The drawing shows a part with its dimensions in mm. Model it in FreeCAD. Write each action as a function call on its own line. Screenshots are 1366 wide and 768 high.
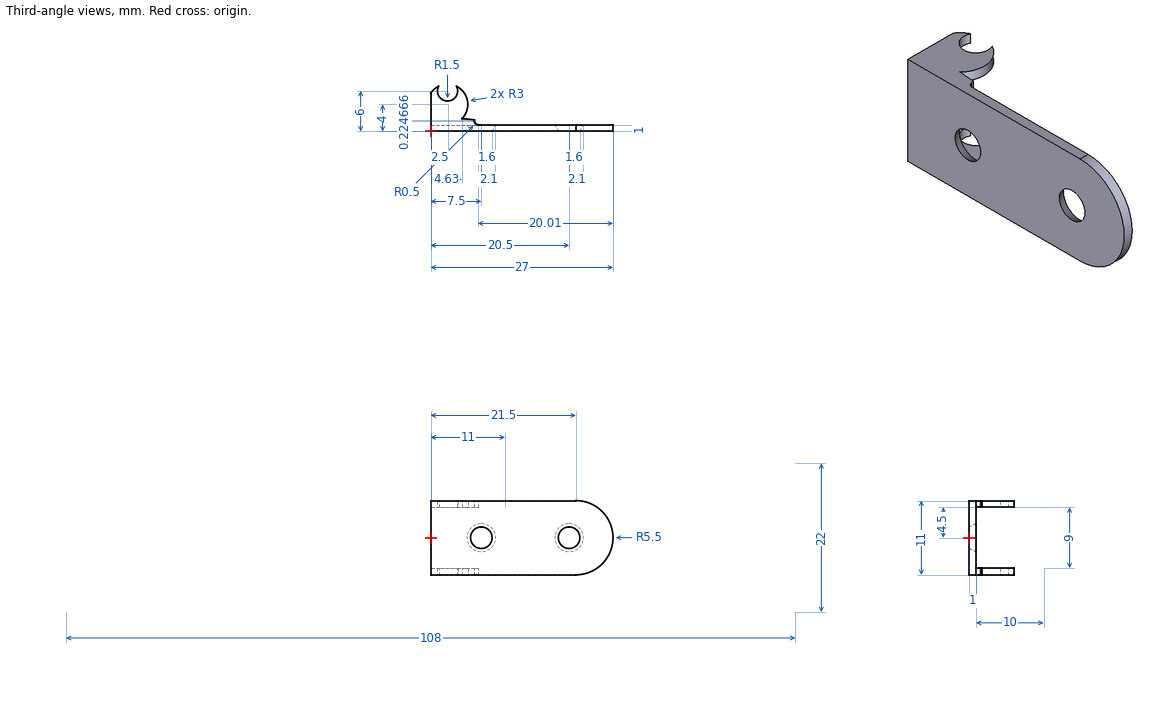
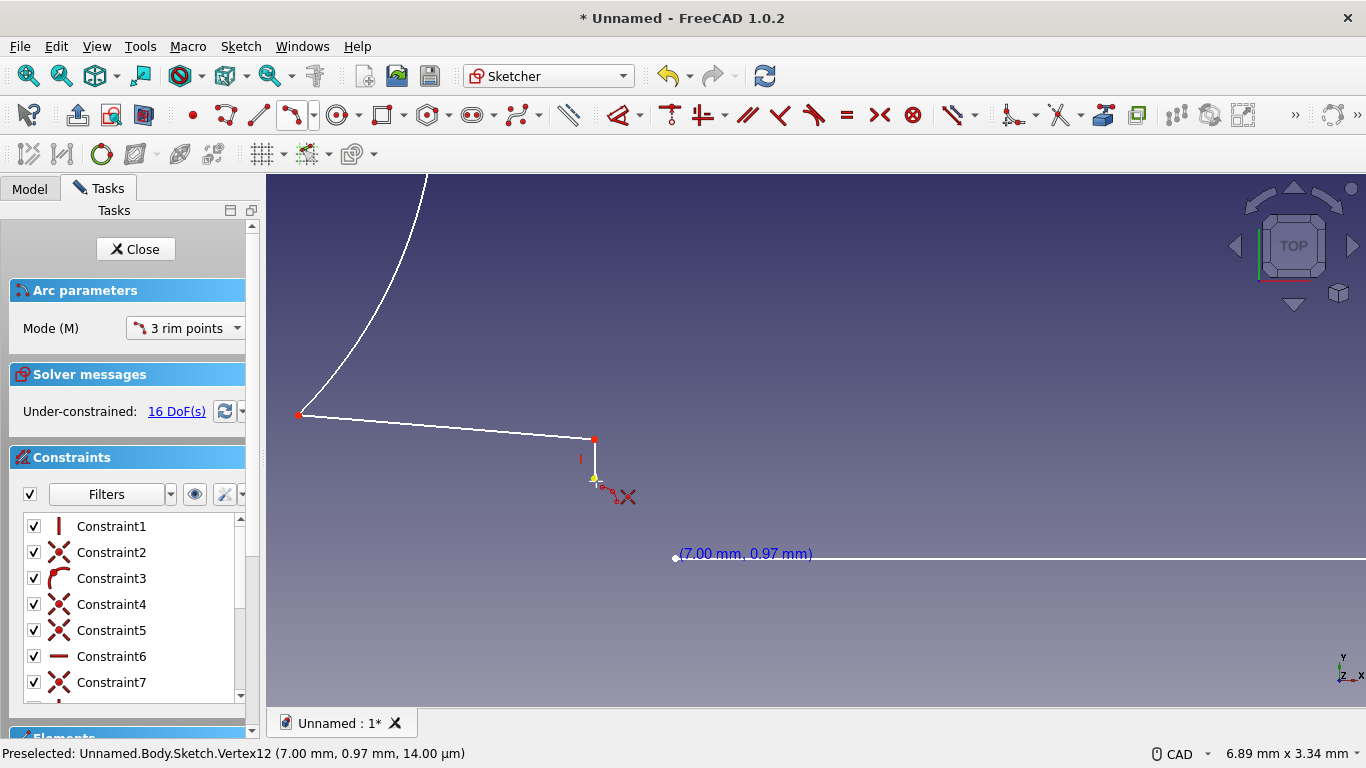
click(595, 478)
click(618, 531)
key(Escape)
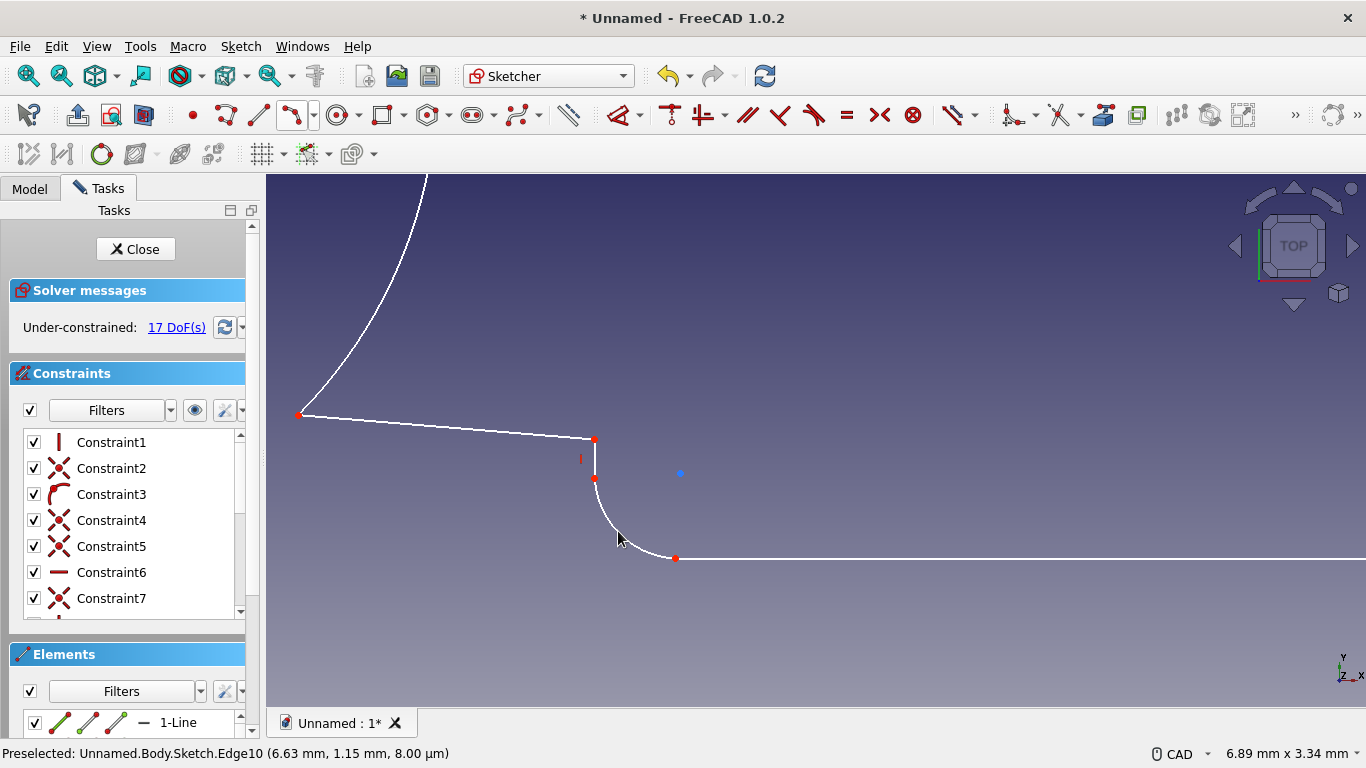
click(595, 467)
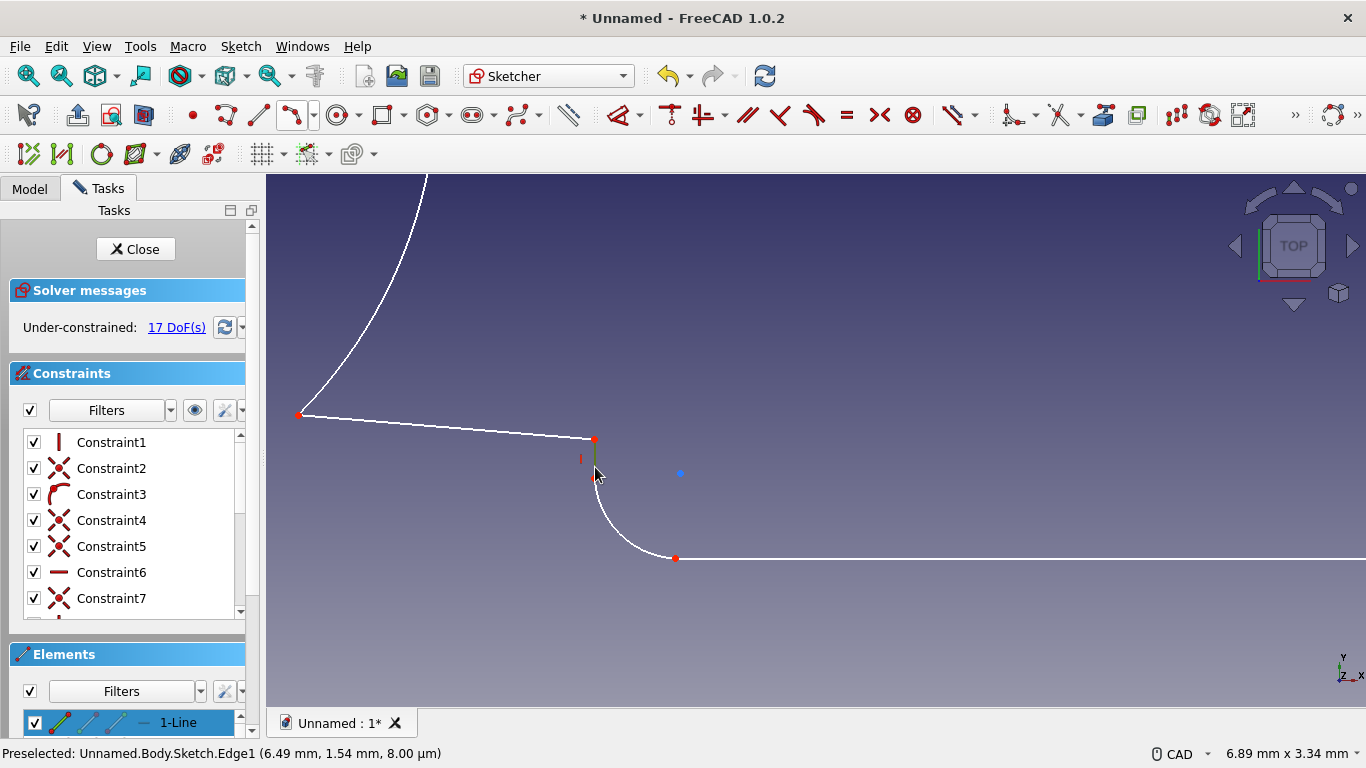
click(605, 514)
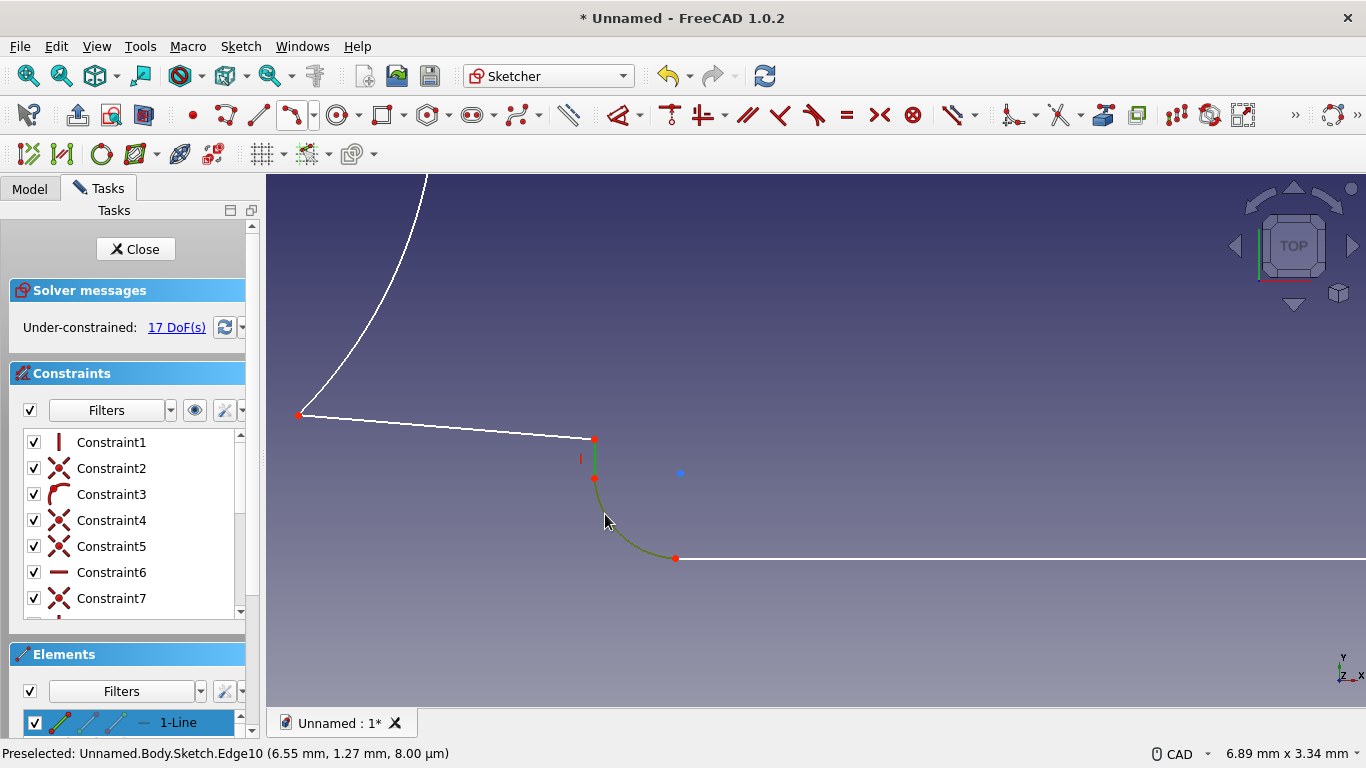
key(t)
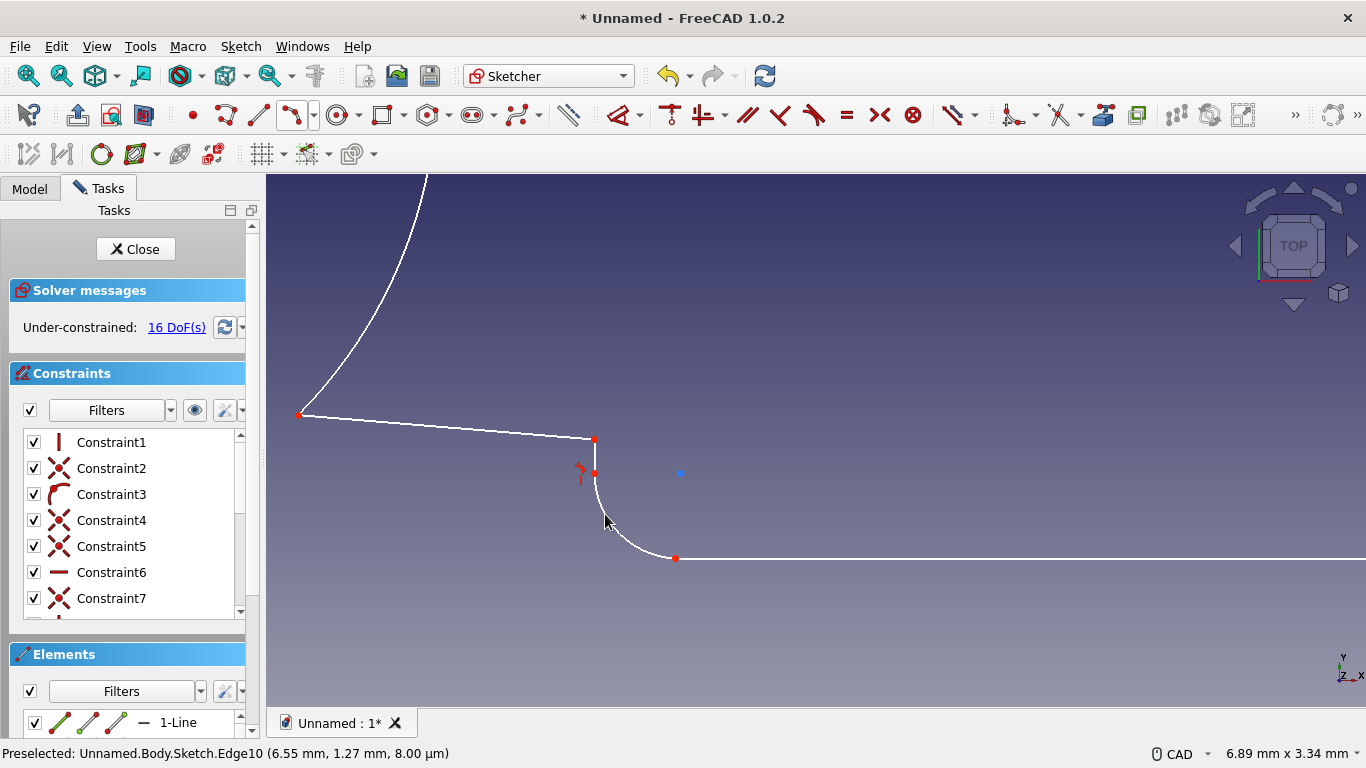
scroll(596, 481, down, 10)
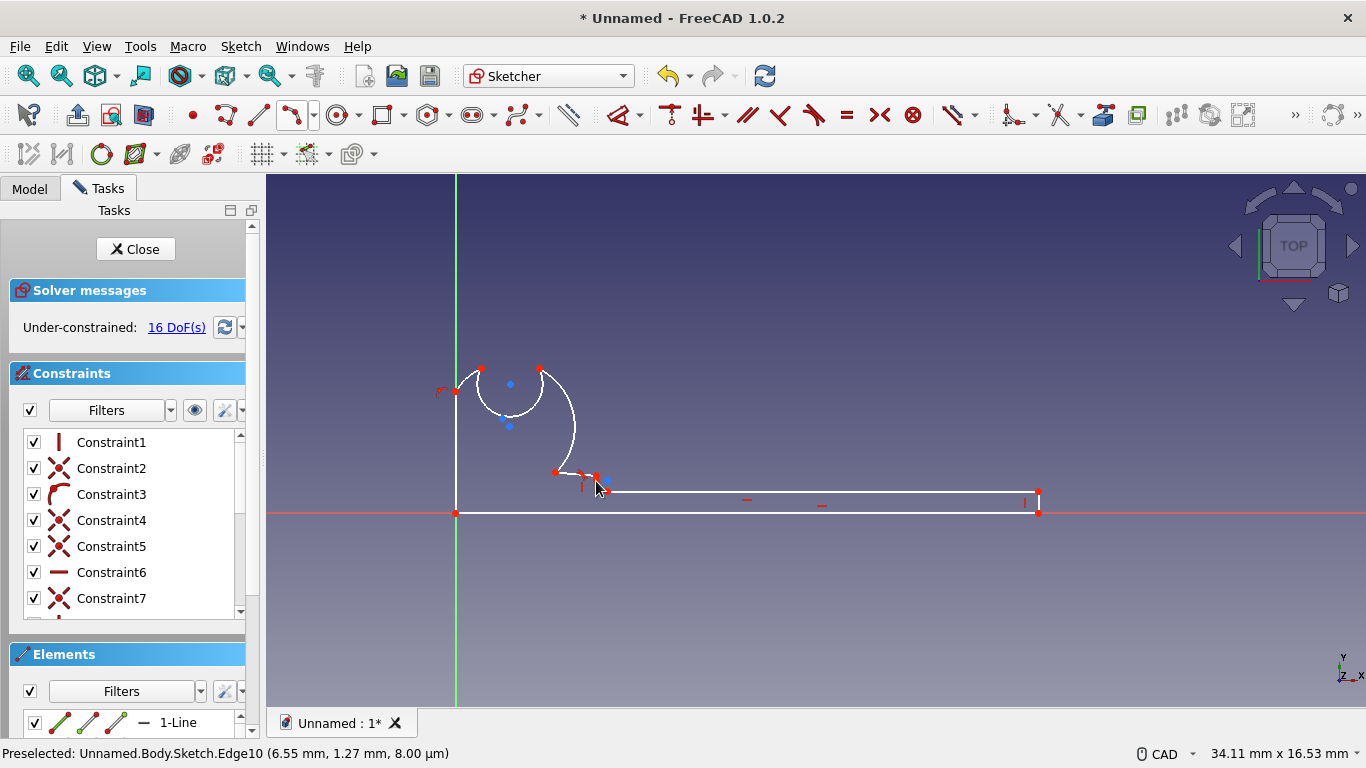
click(909, 492)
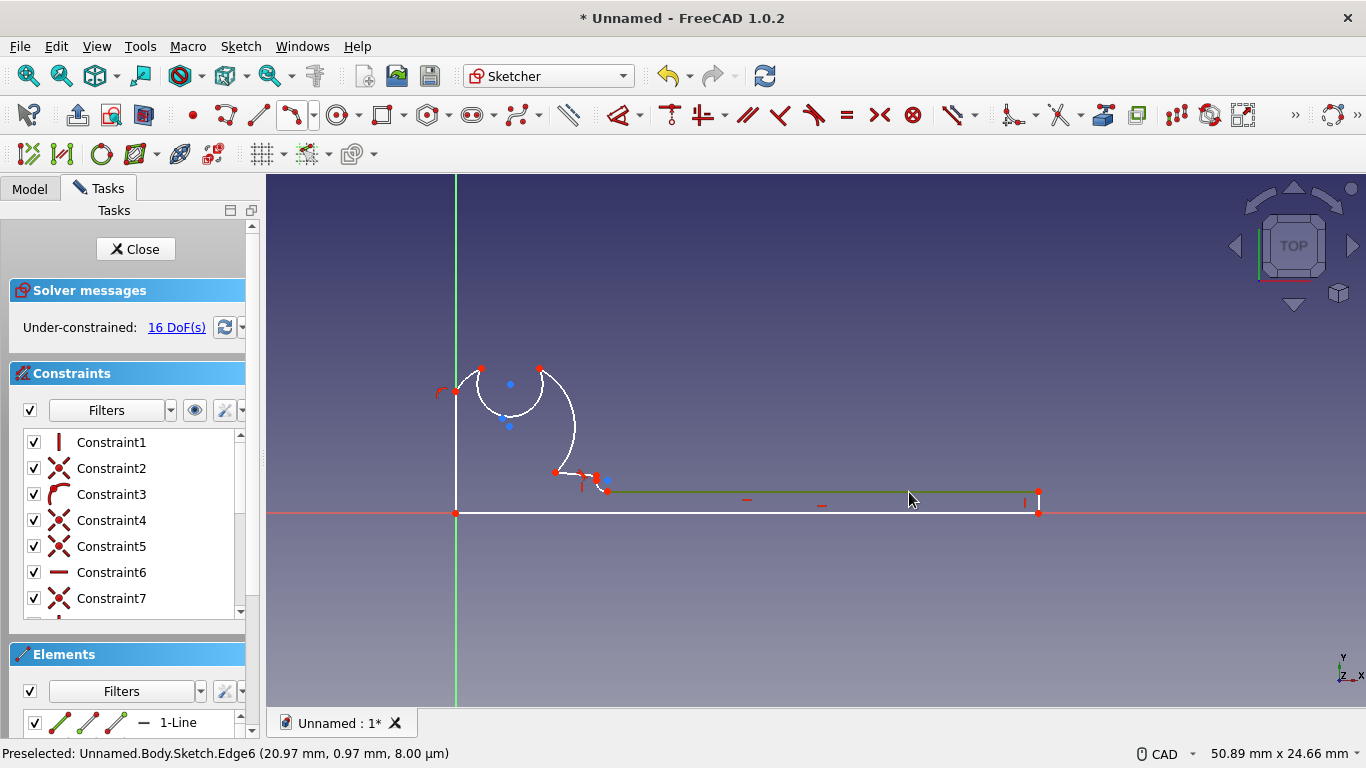
scroll(599, 488, up, 3)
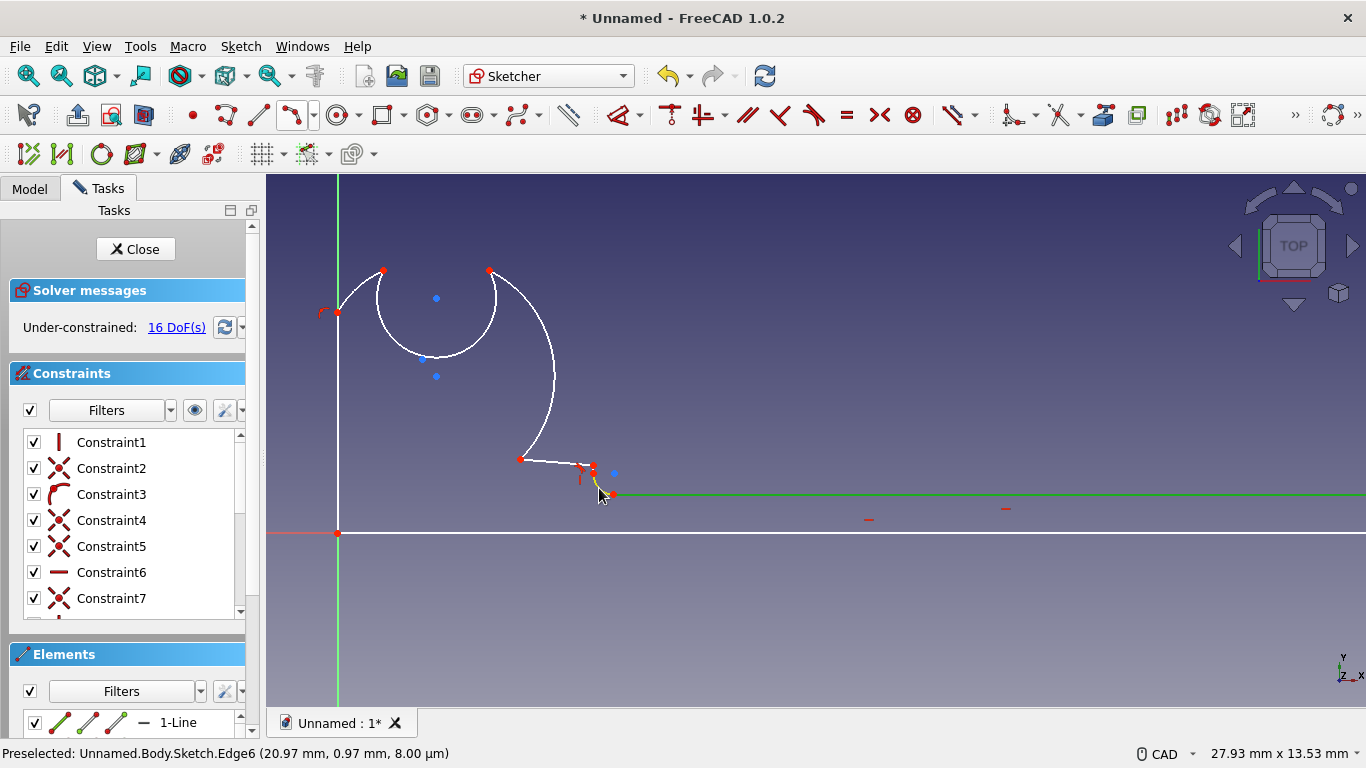
click(599, 488)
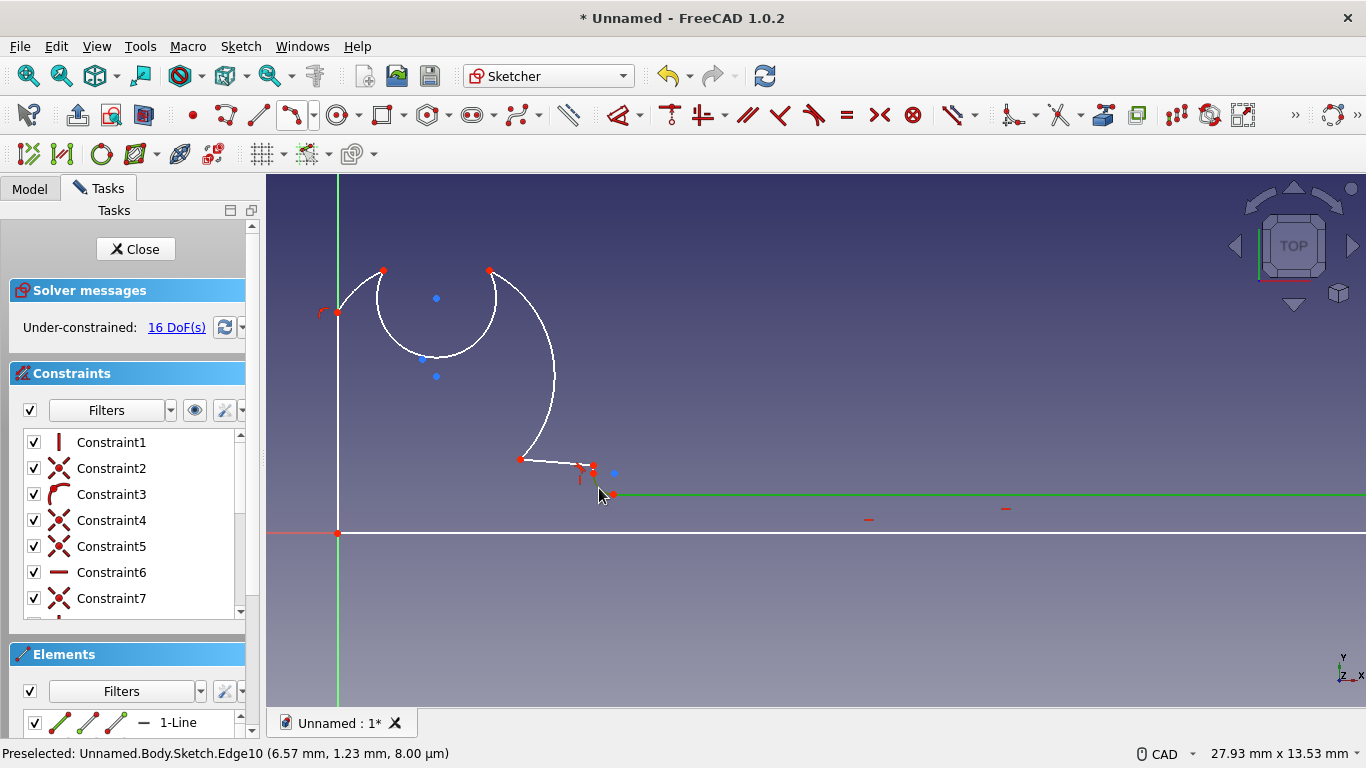
key(t)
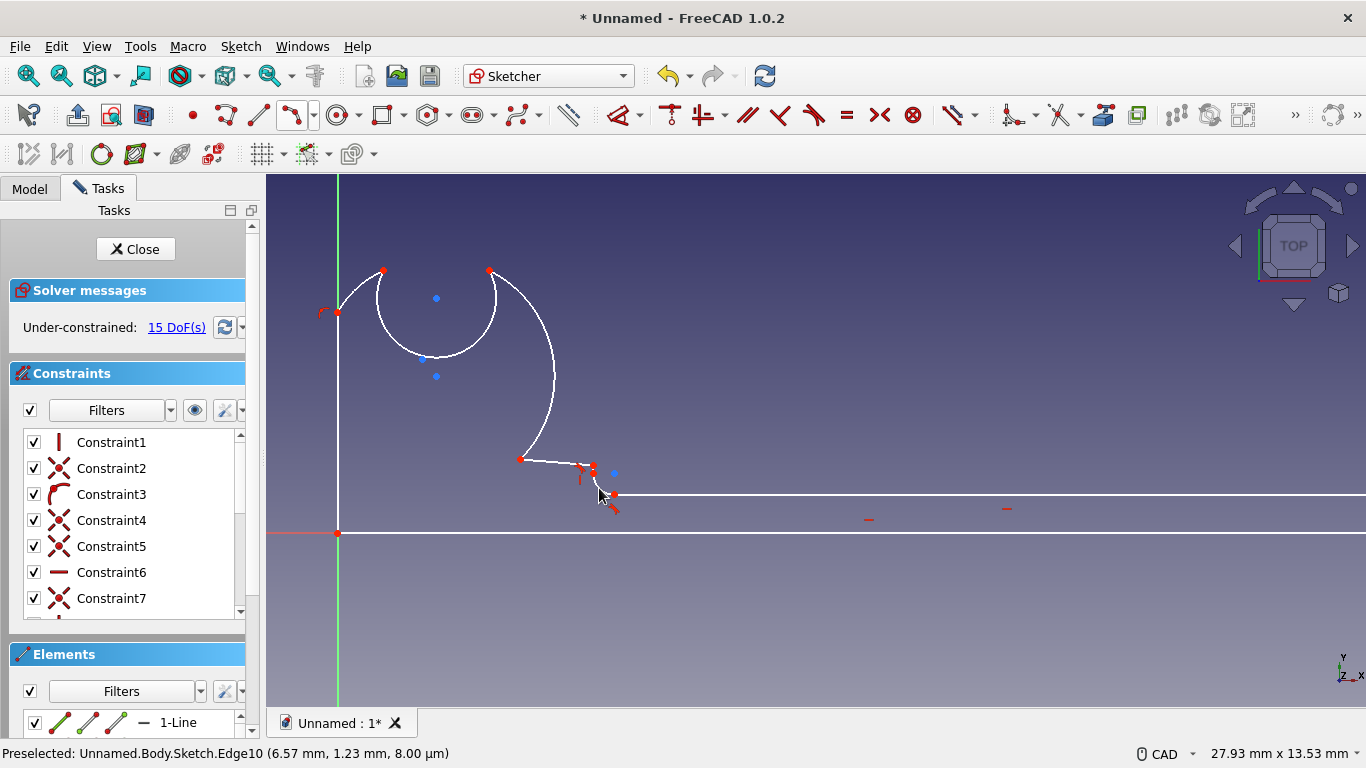
click(552, 401)